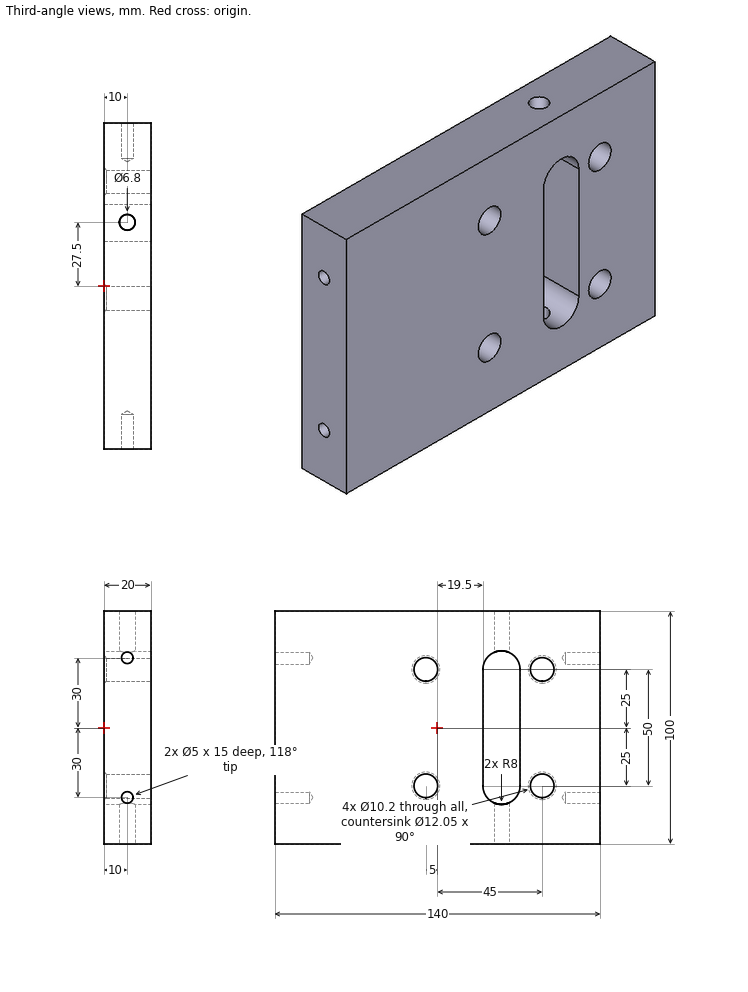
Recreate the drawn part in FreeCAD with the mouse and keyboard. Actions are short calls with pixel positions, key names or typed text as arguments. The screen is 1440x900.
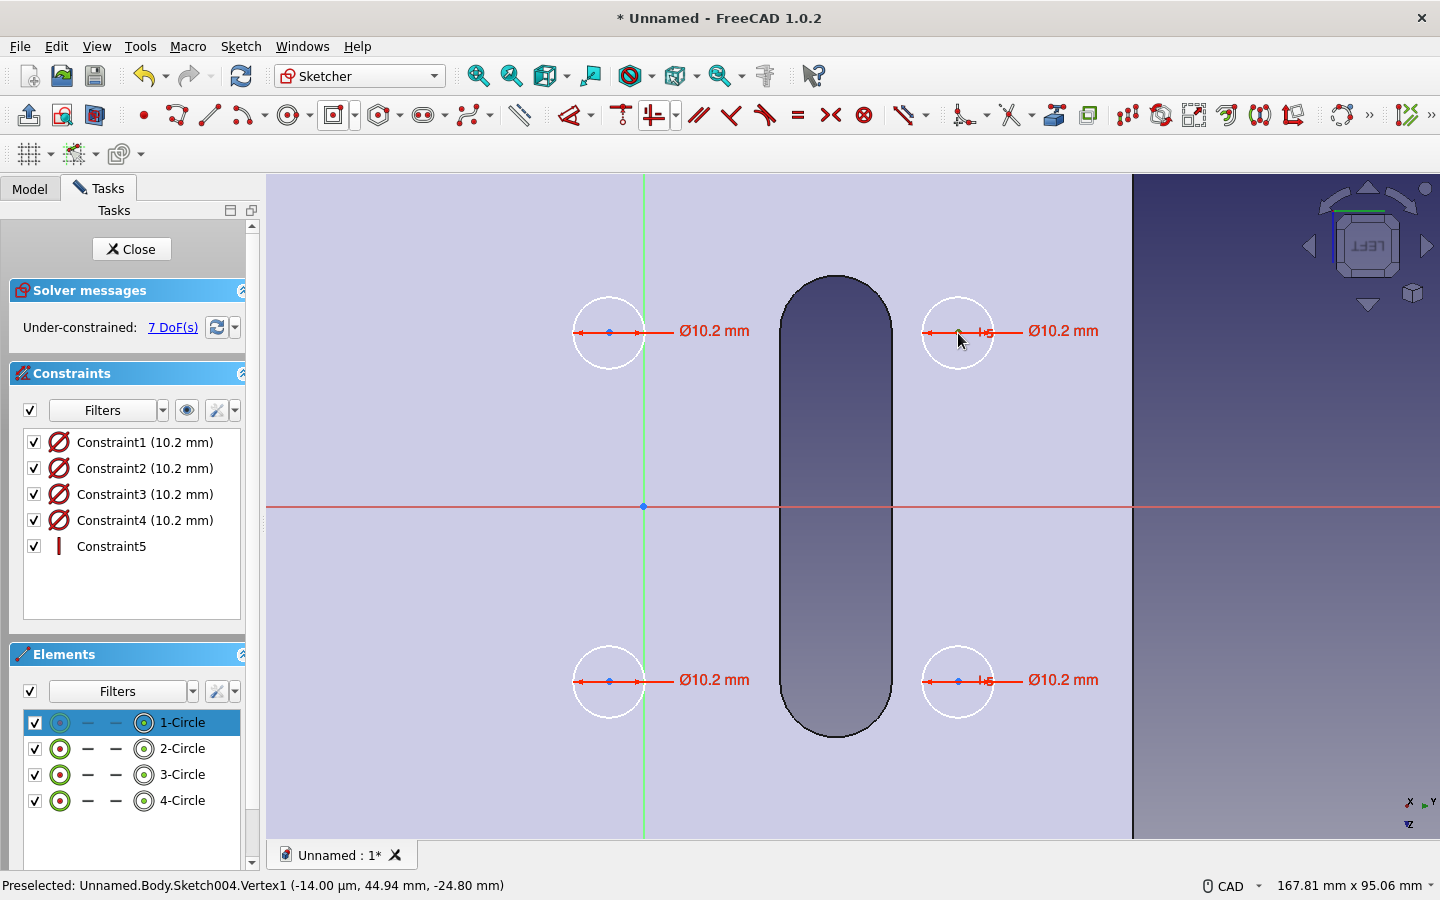
click(609, 333)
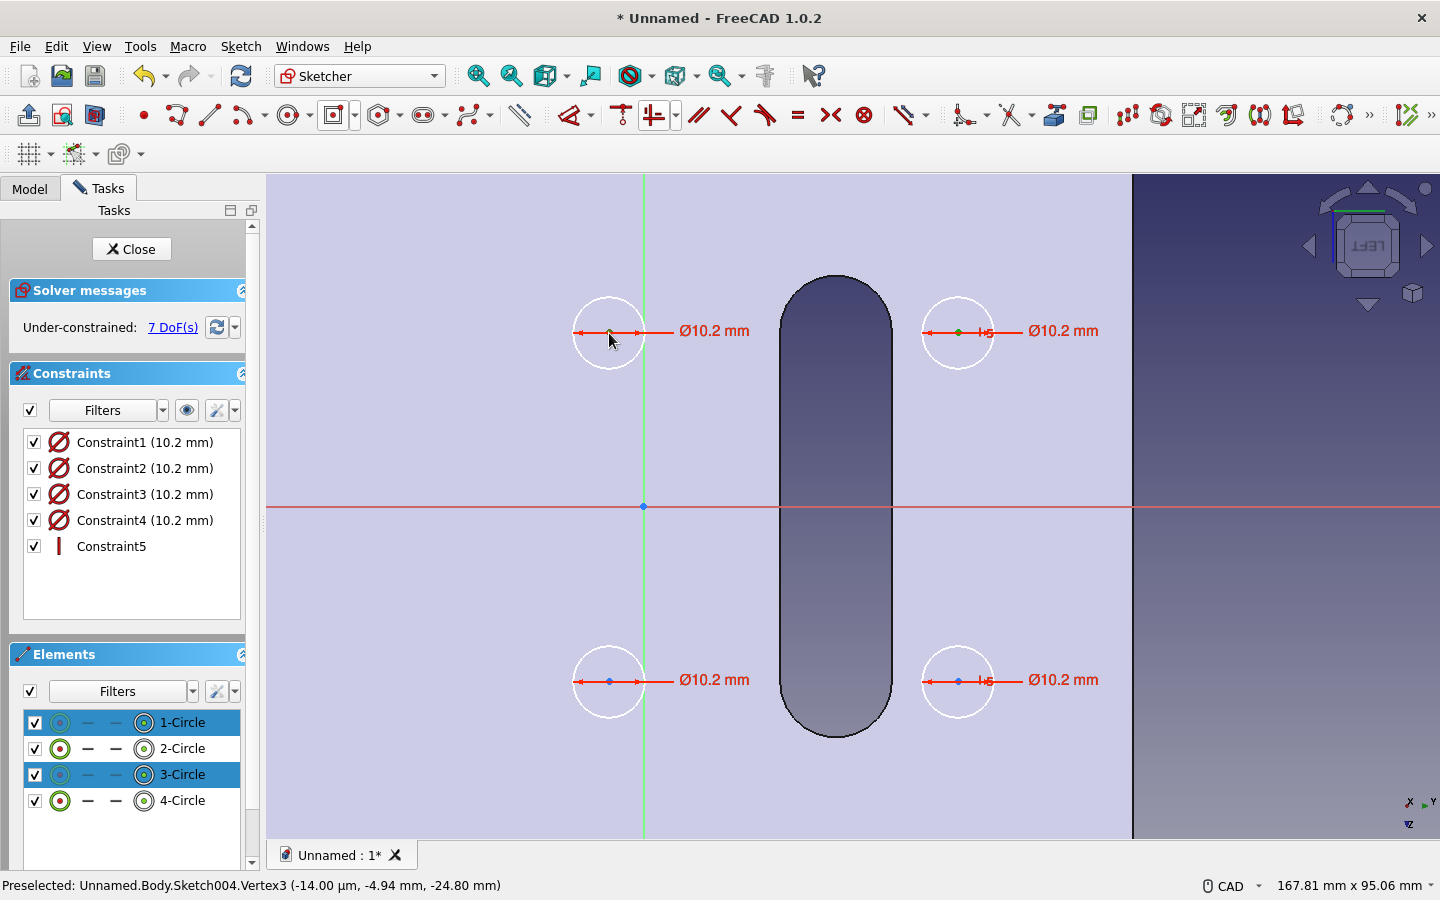
click(676, 116)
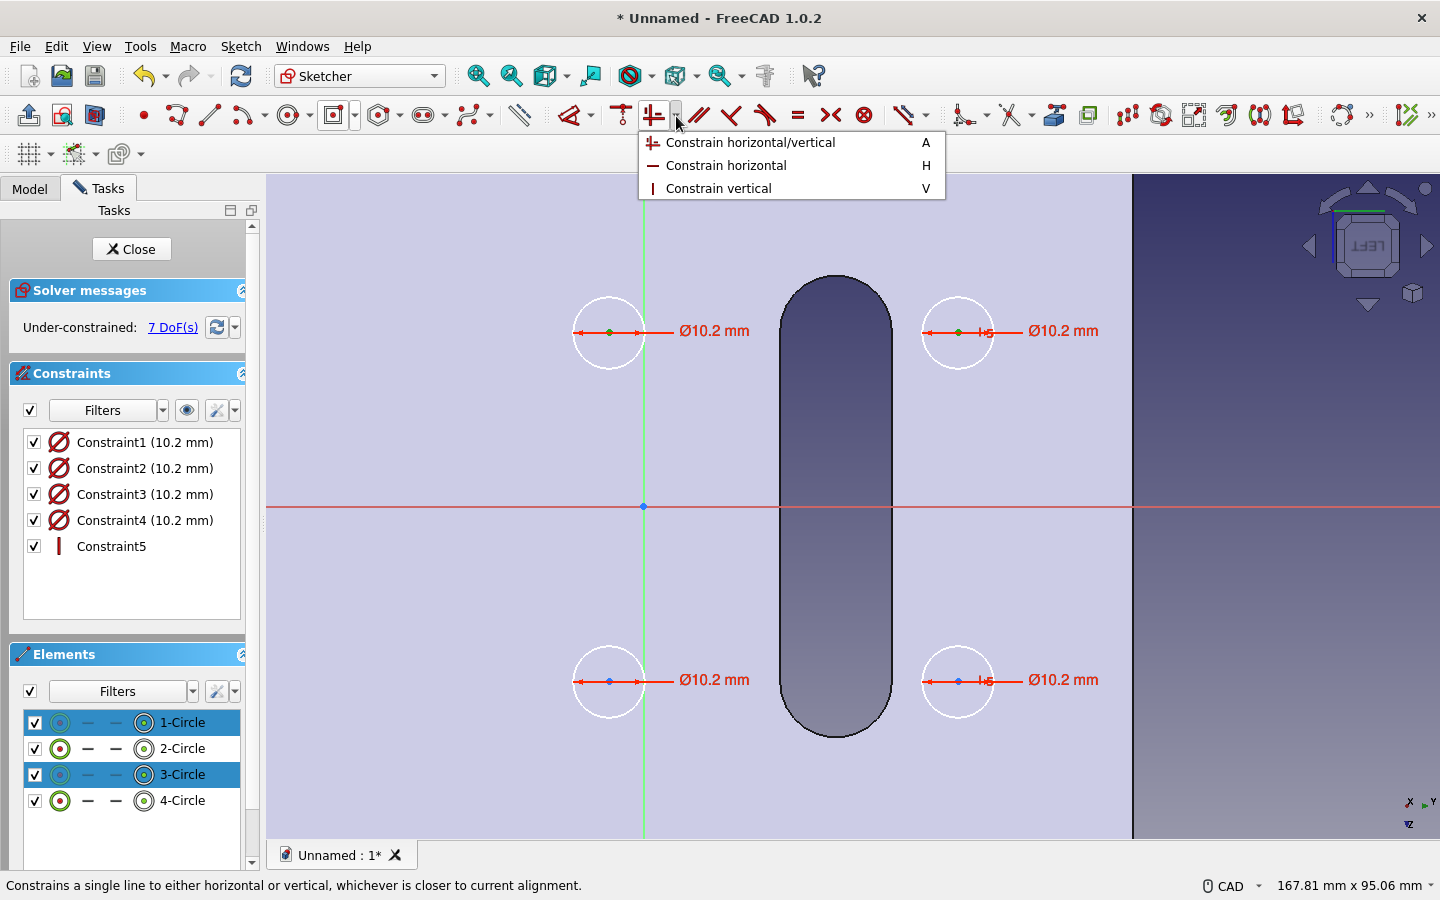
click(792, 166)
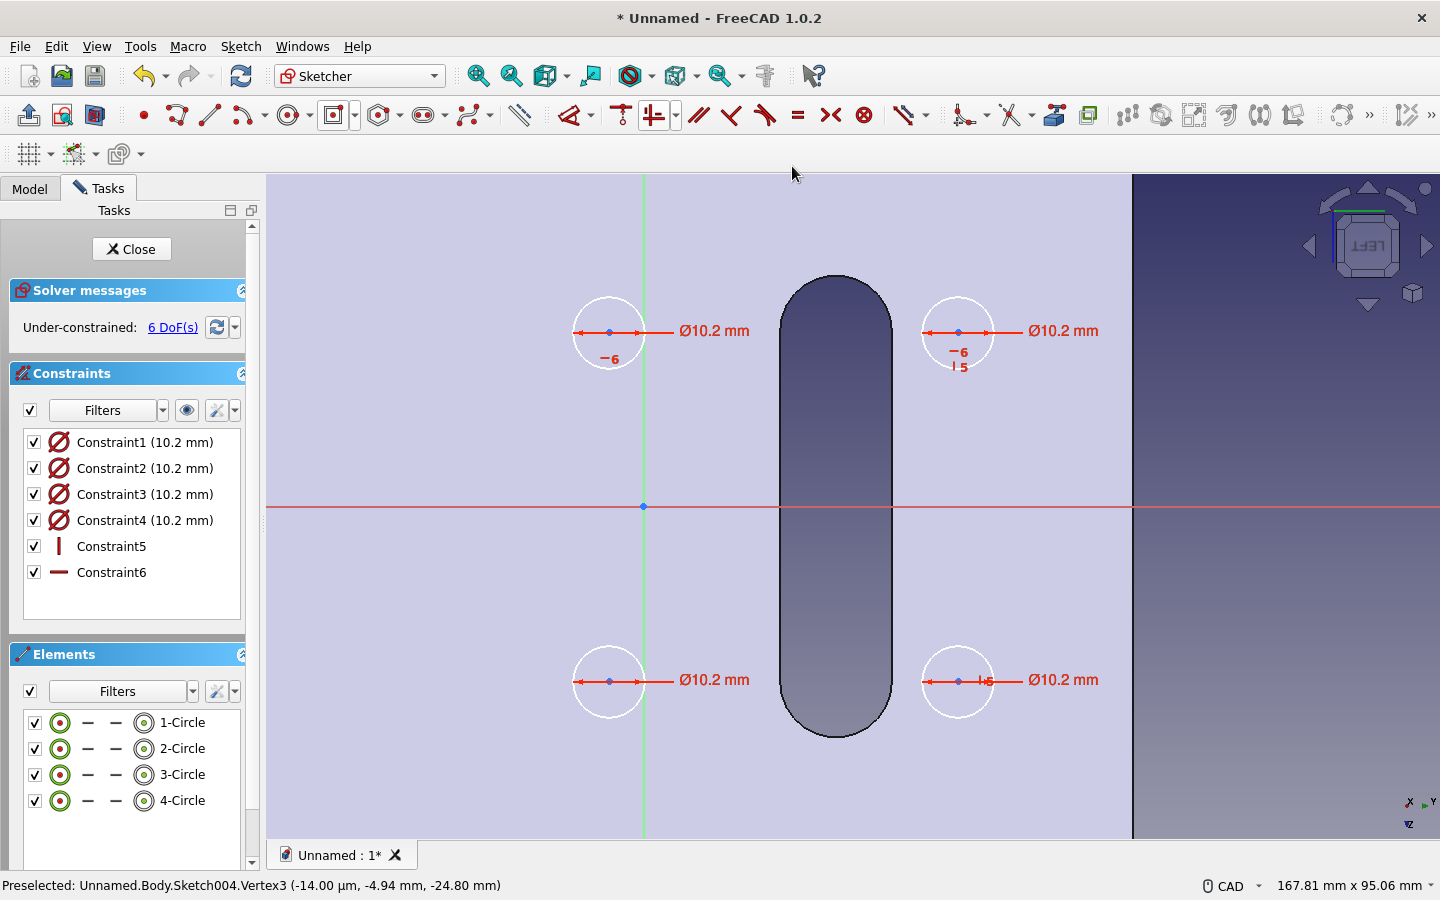
click(609, 333)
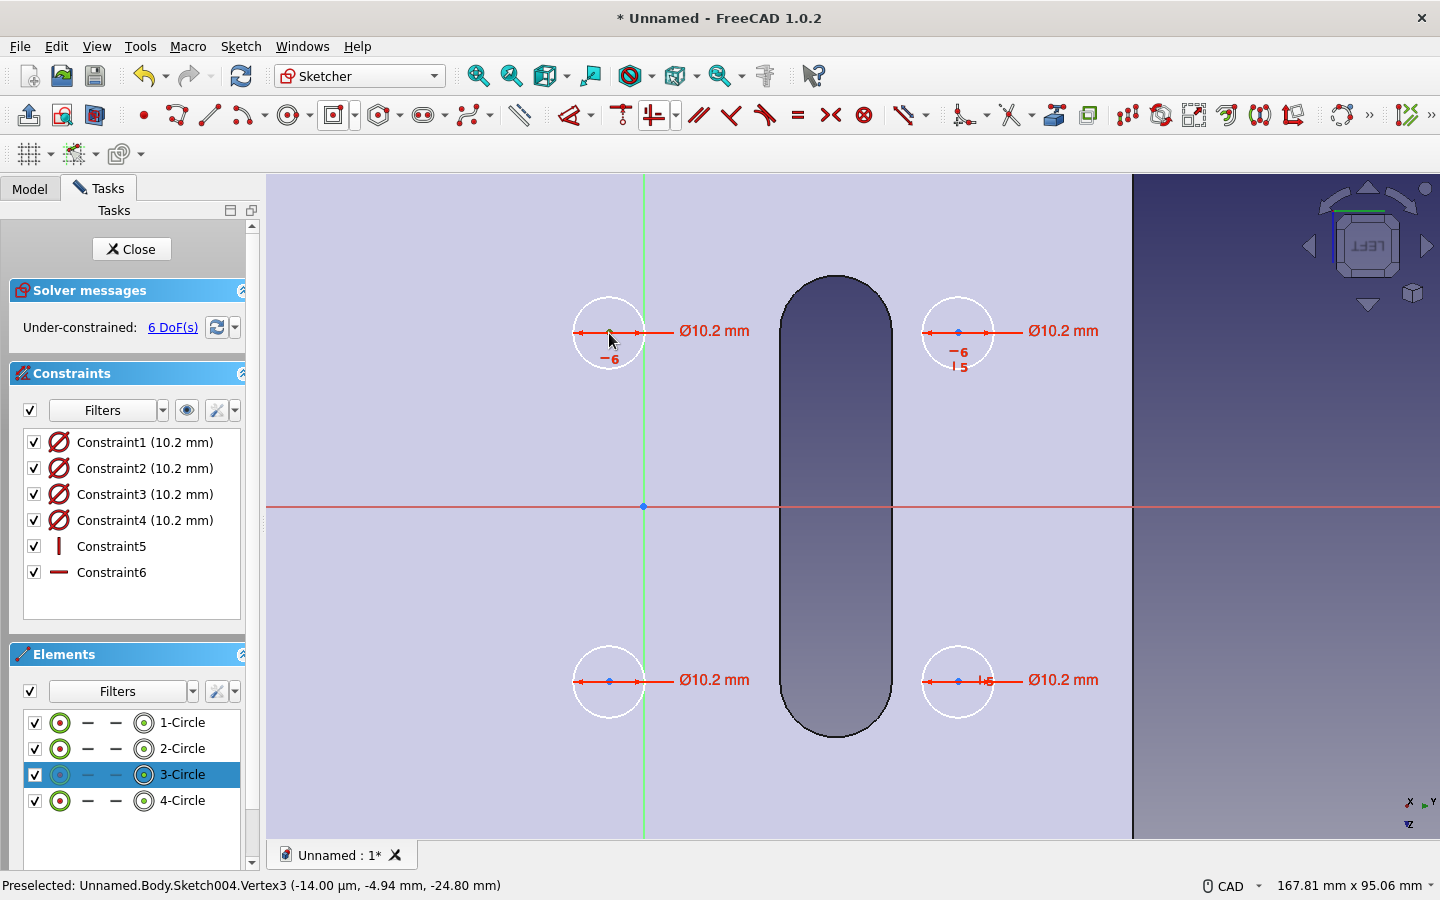
click(609, 682)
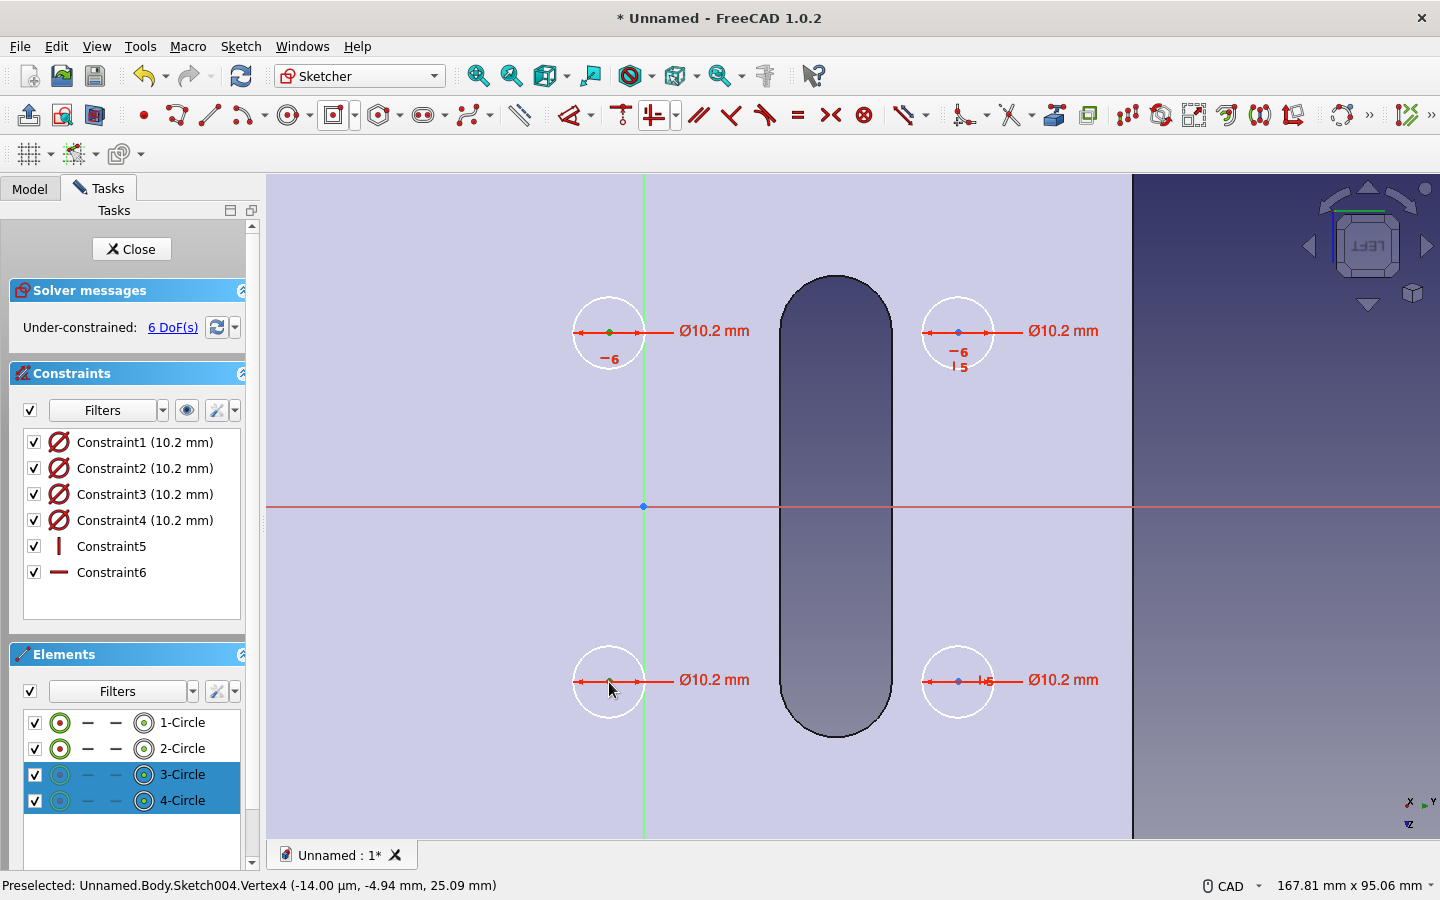
click(676, 116)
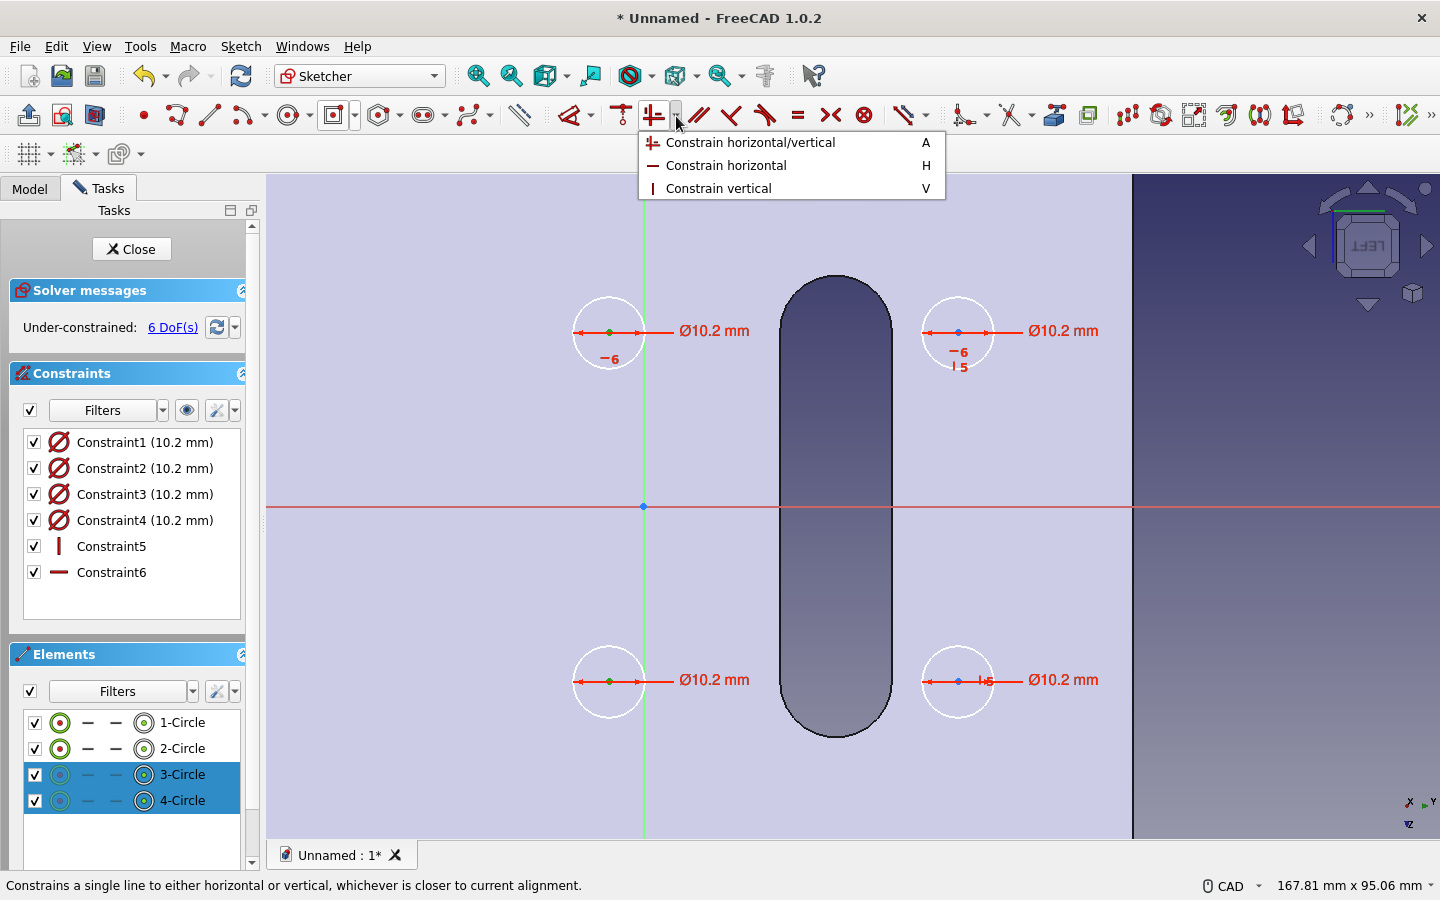
click(792, 188)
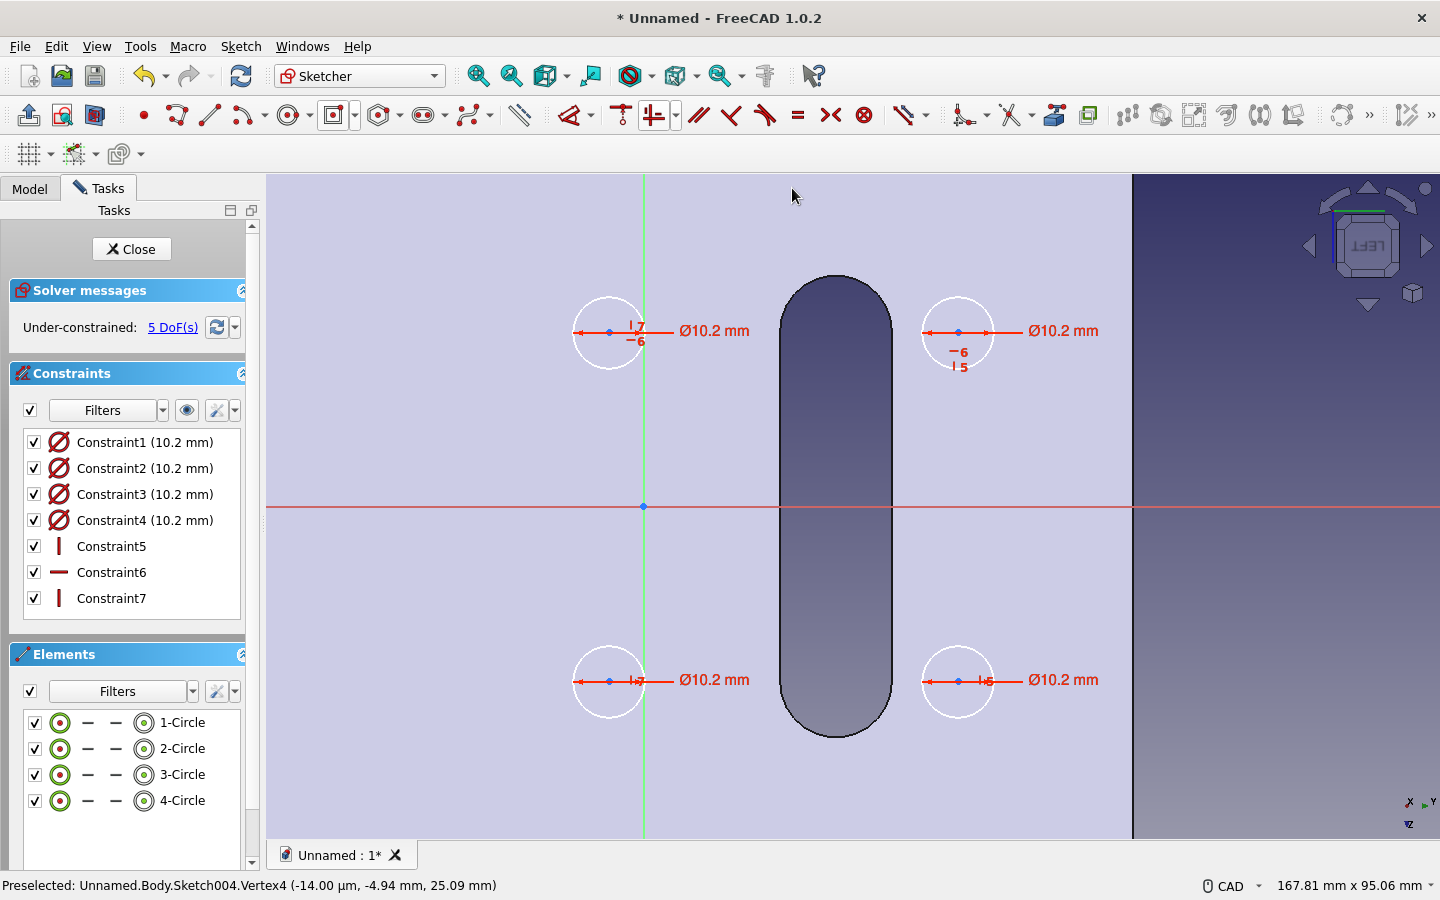
click(958, 682)